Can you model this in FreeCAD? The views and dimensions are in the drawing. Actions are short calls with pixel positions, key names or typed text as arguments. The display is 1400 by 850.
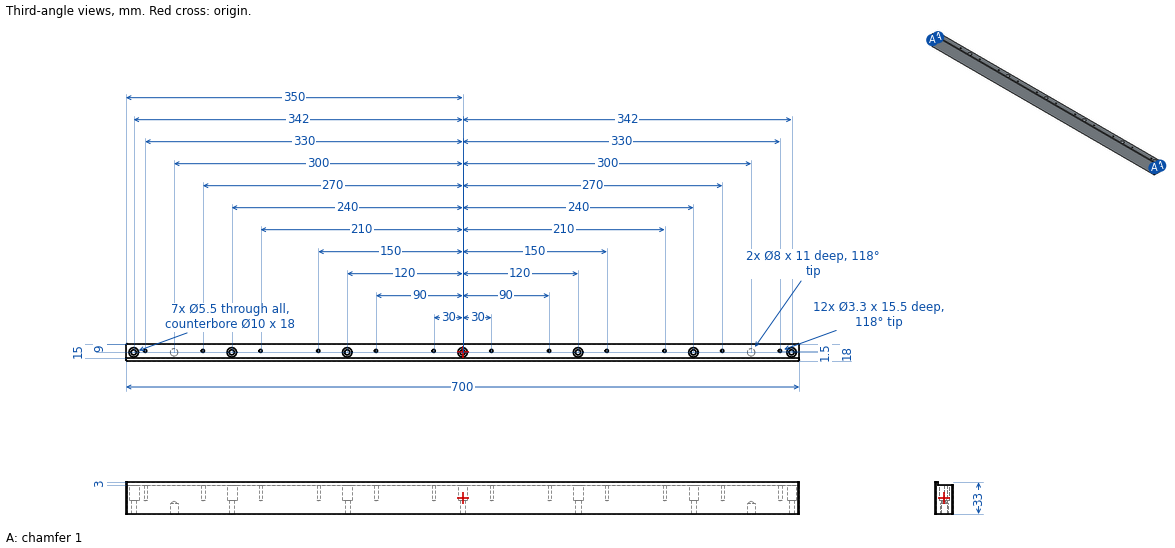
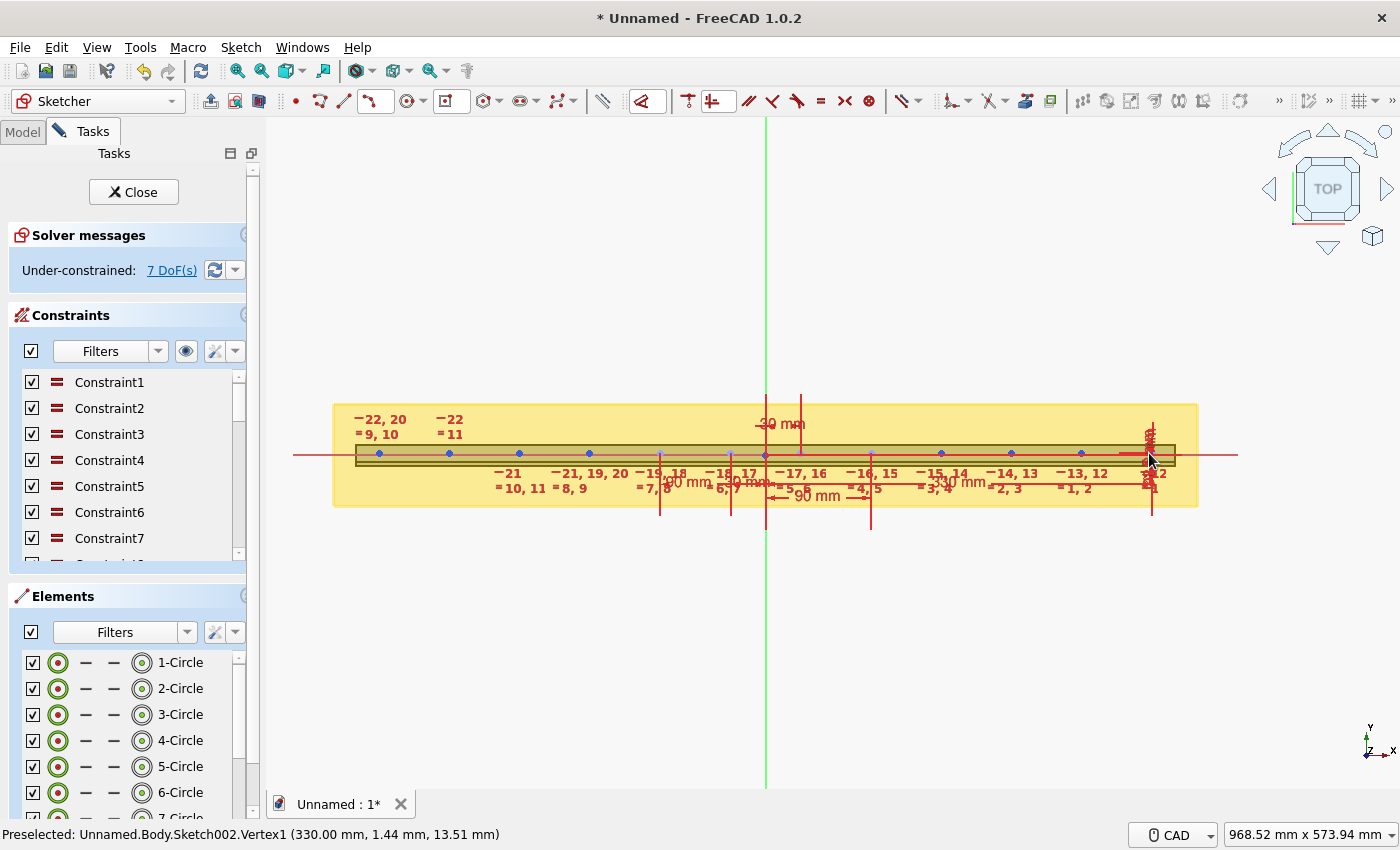
click(1082, 453)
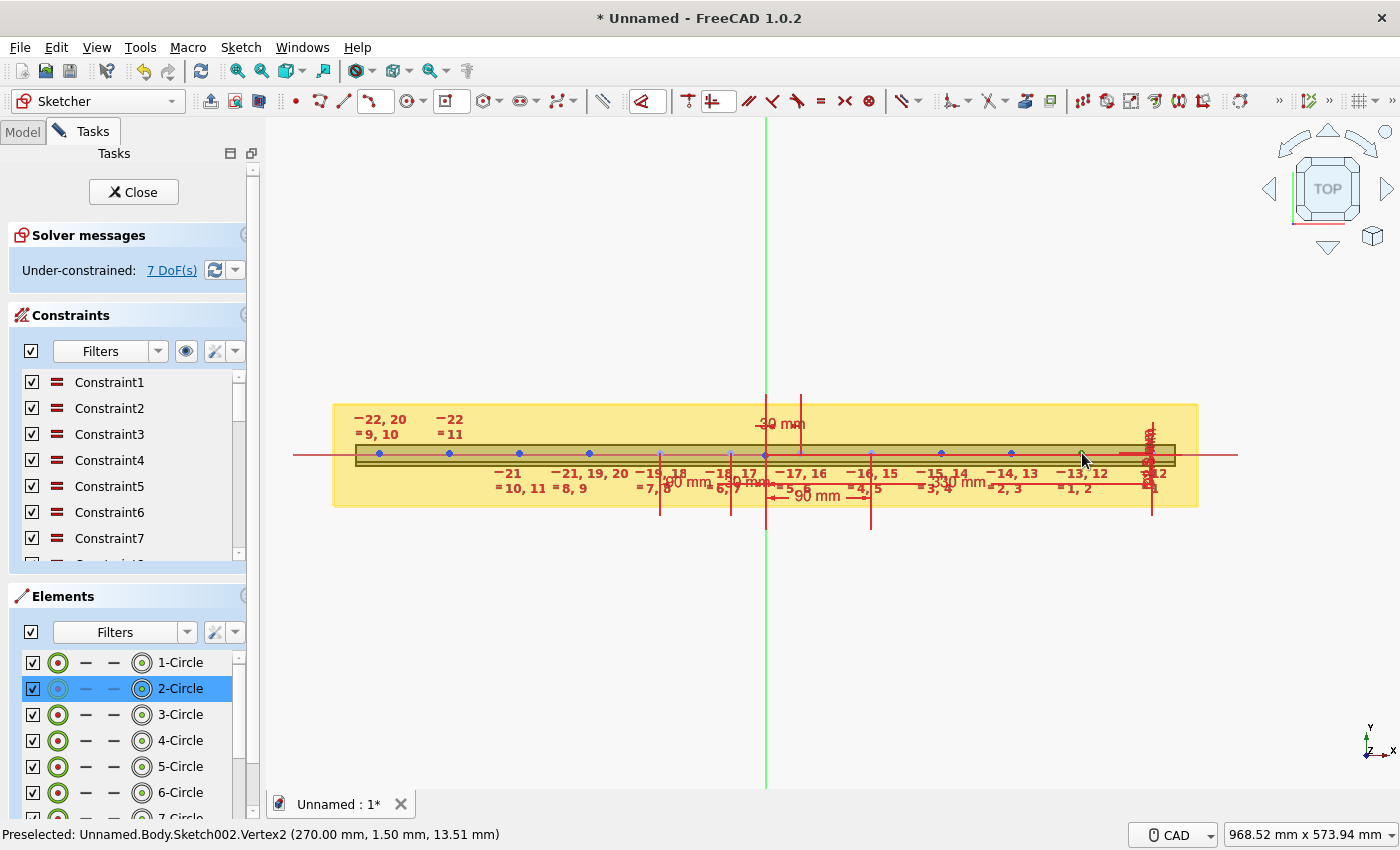
key(l)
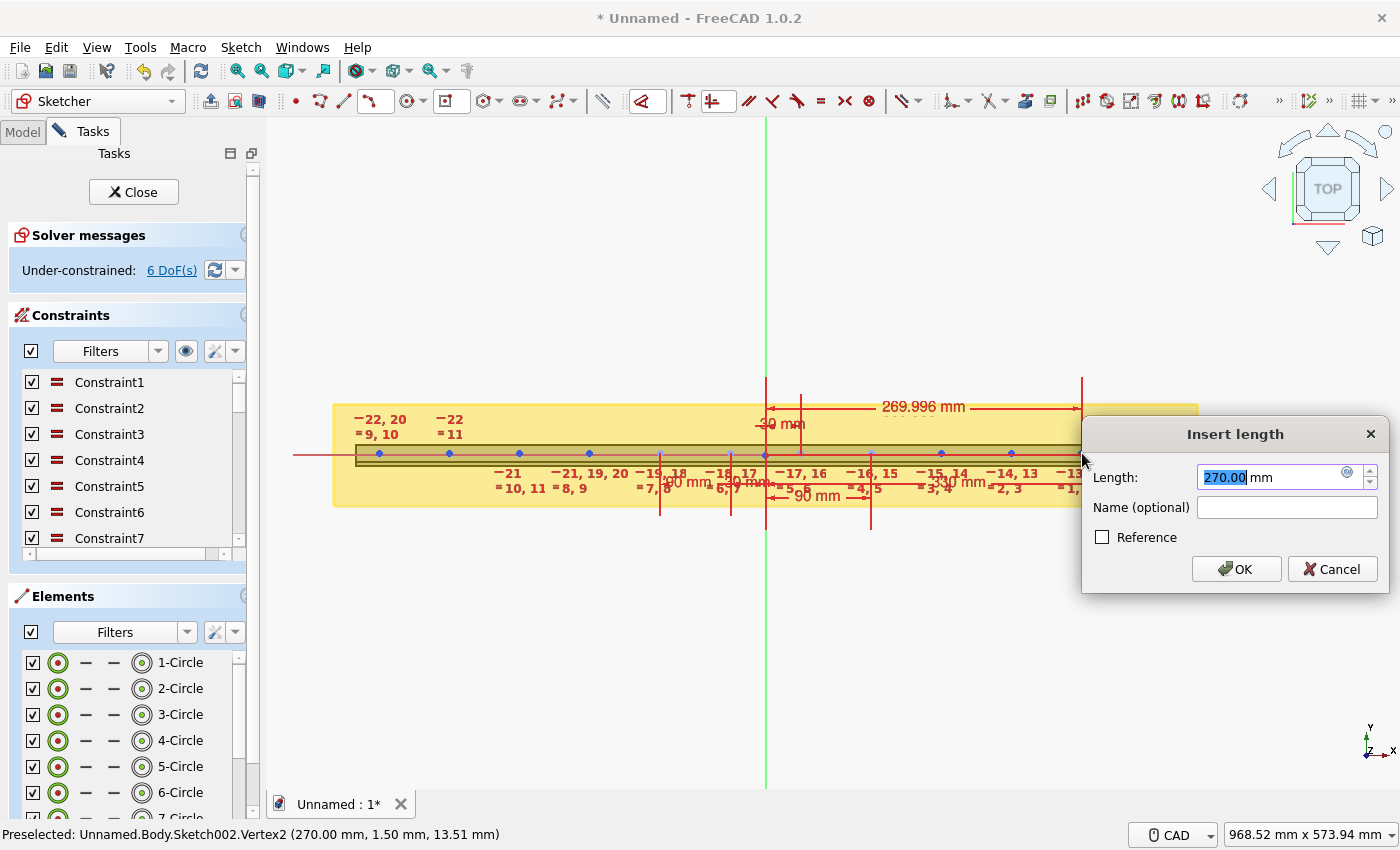
text(270)
key(Return)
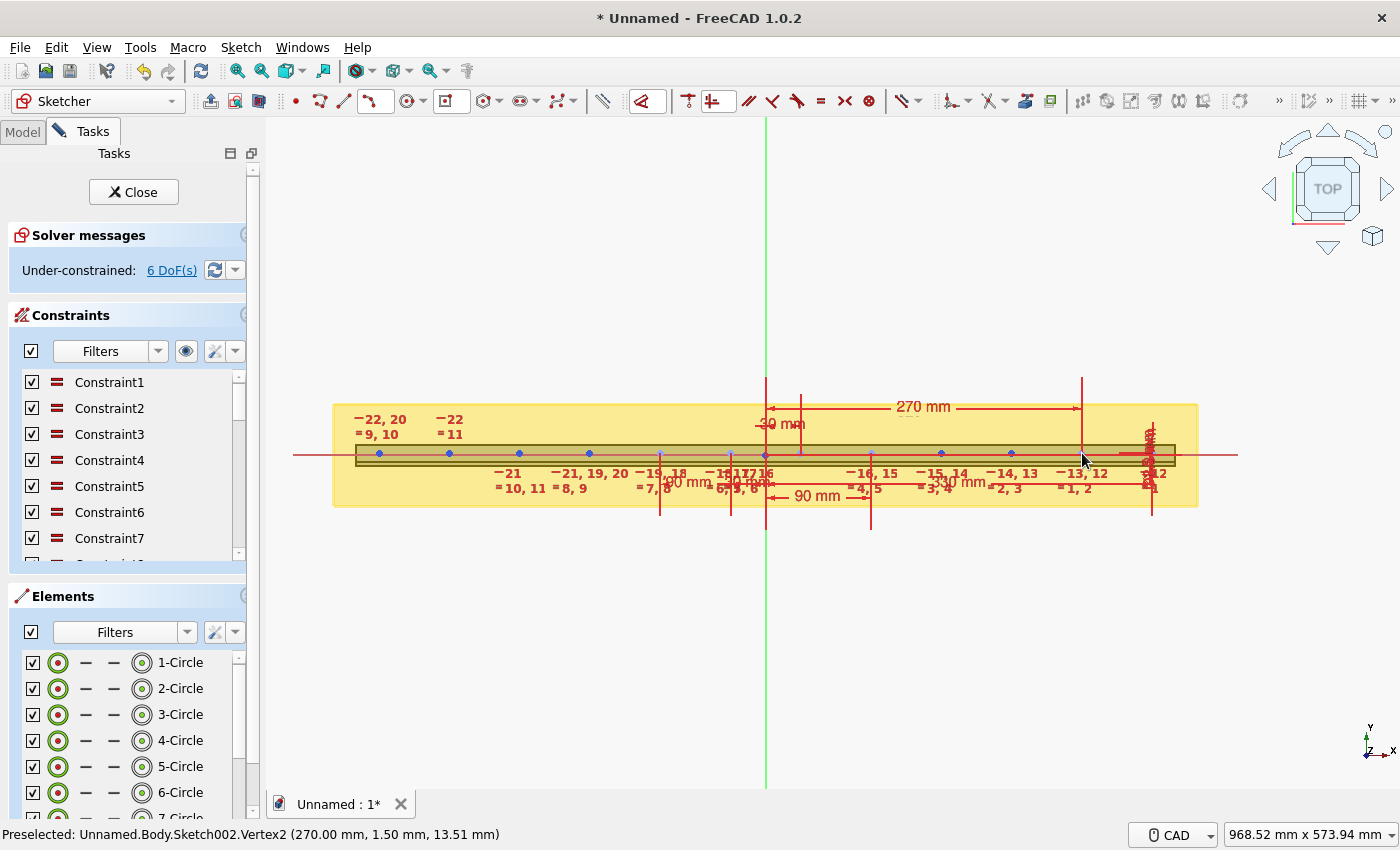
click(1011, 453)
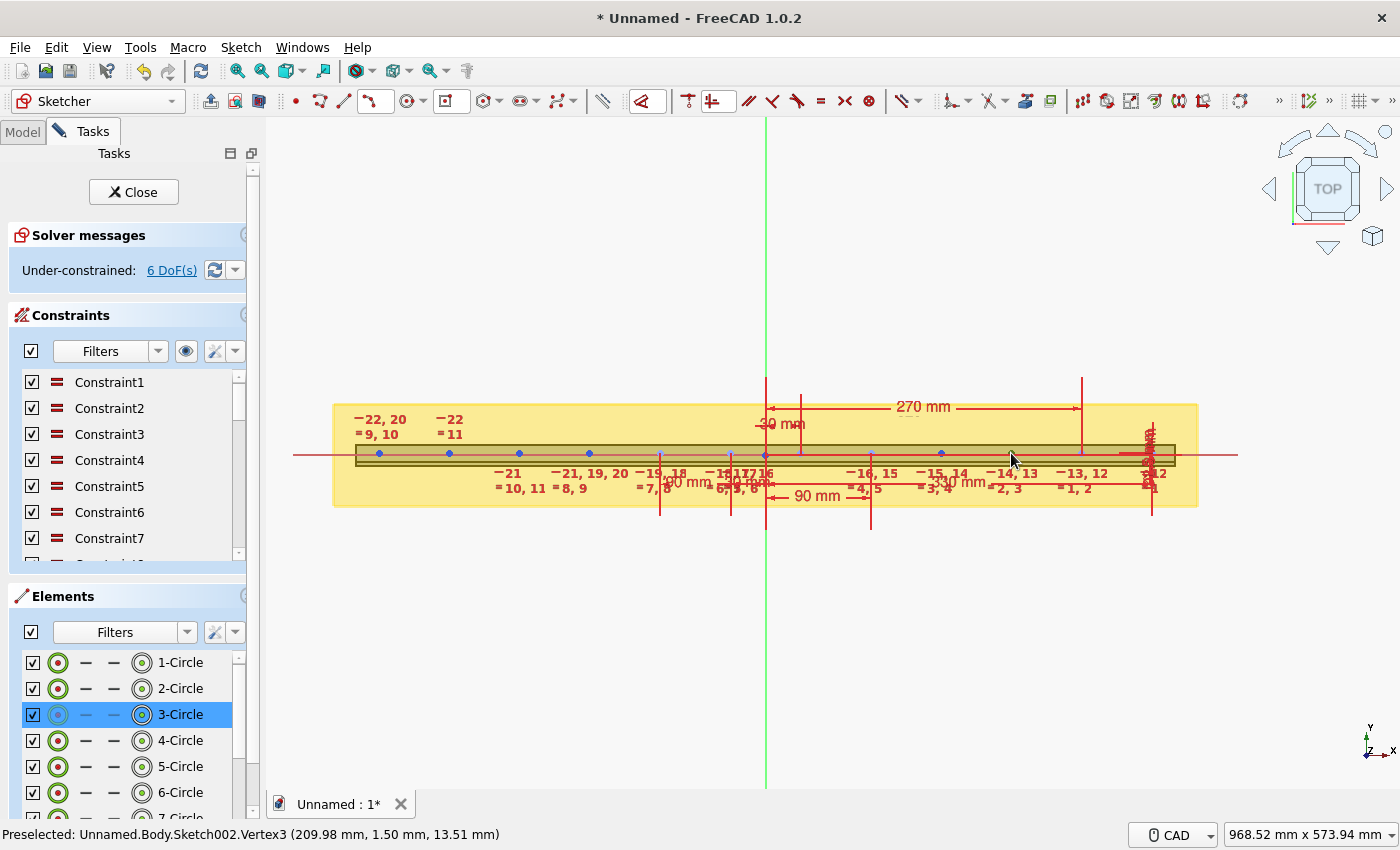
key(l)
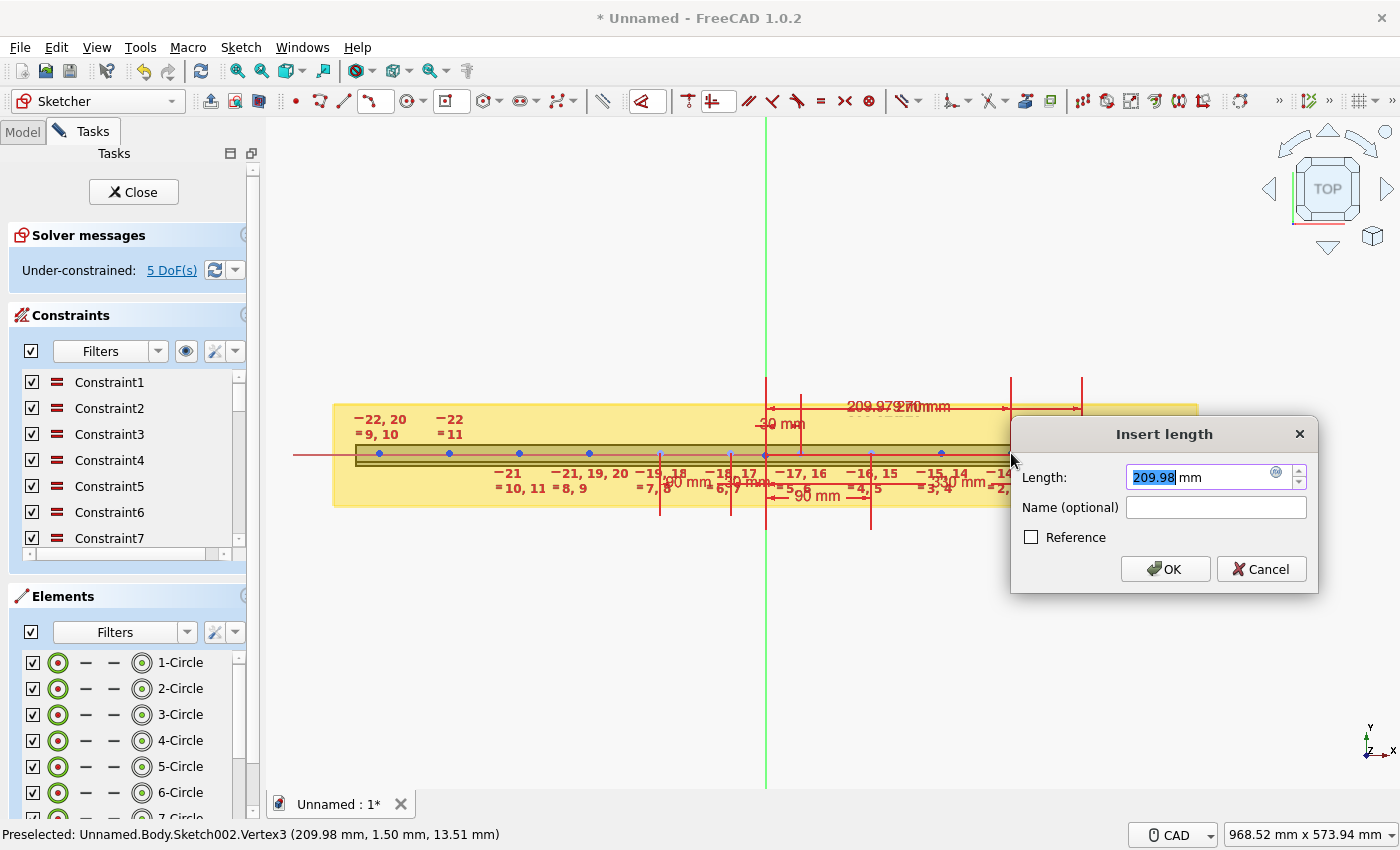
text(210)
key(Return)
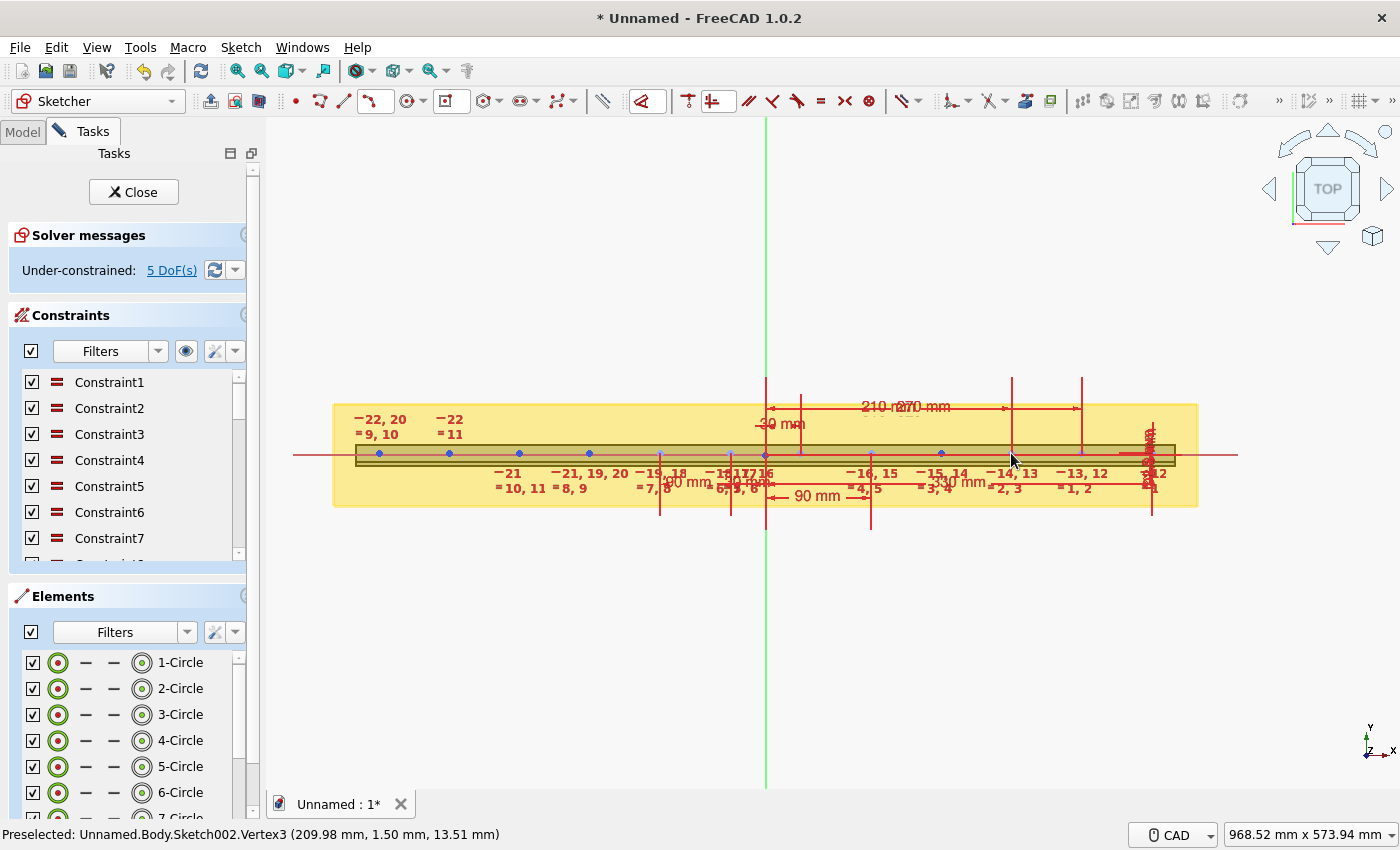
click(941, 453)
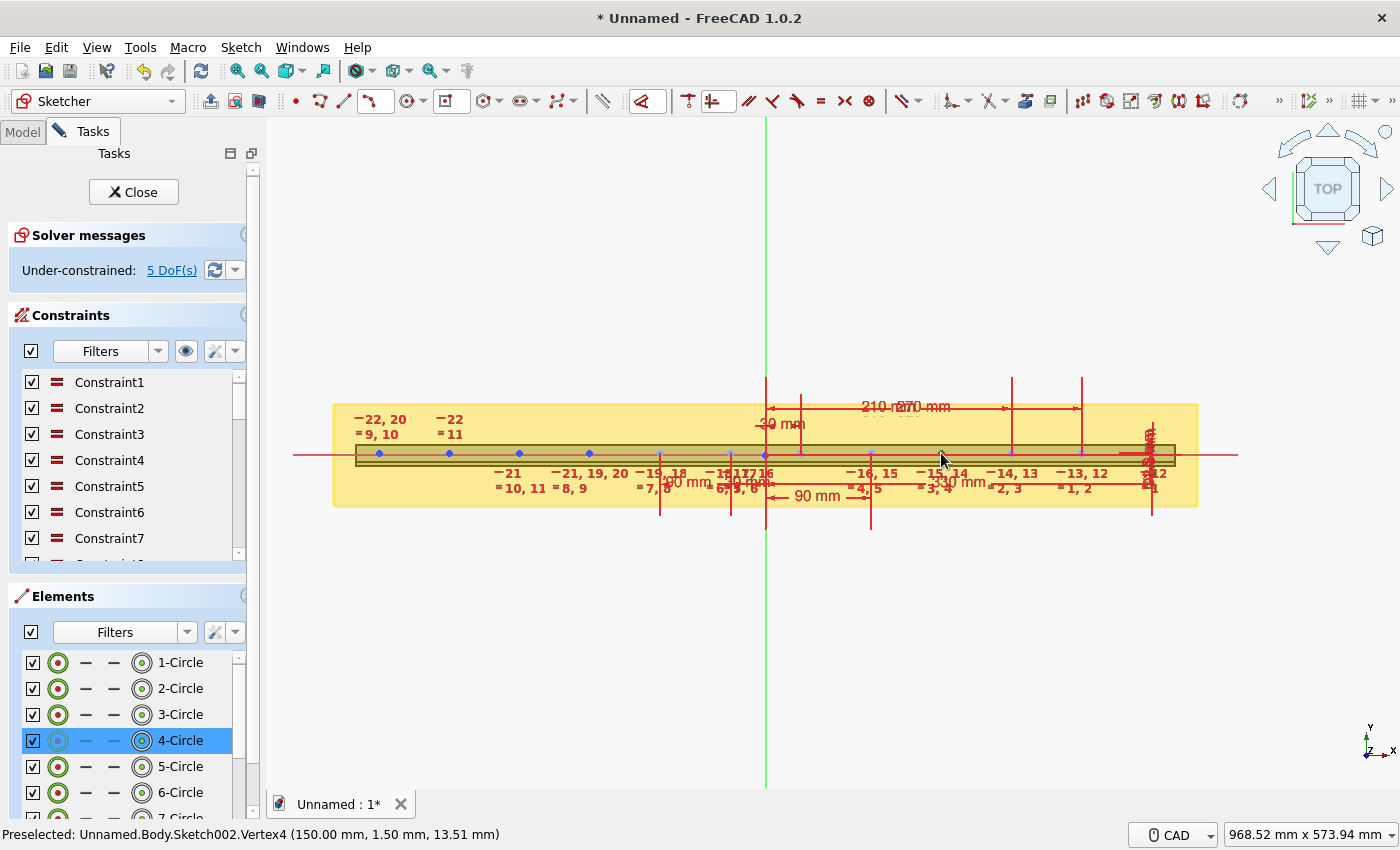
key(l)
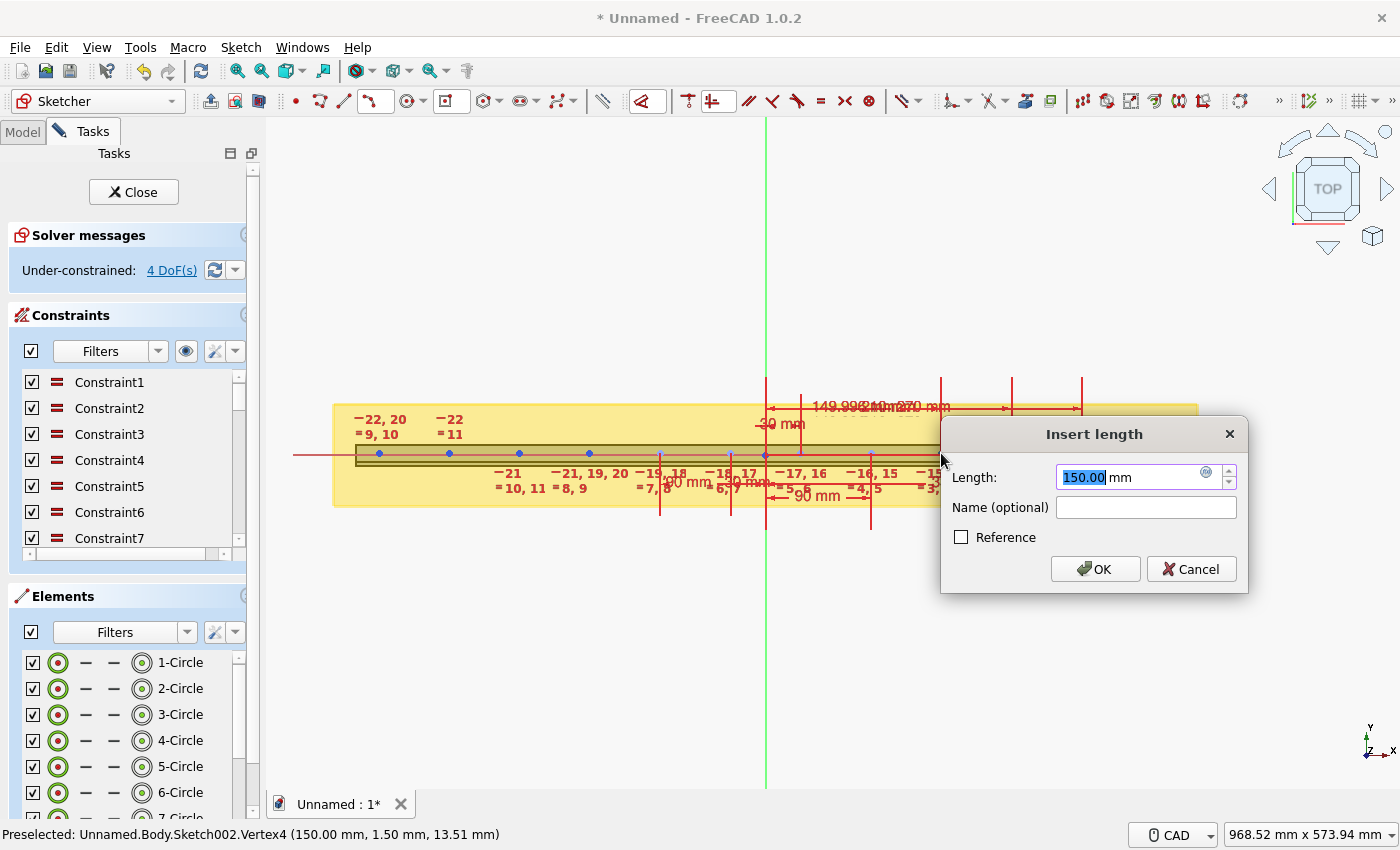
text(150)
key(Return)